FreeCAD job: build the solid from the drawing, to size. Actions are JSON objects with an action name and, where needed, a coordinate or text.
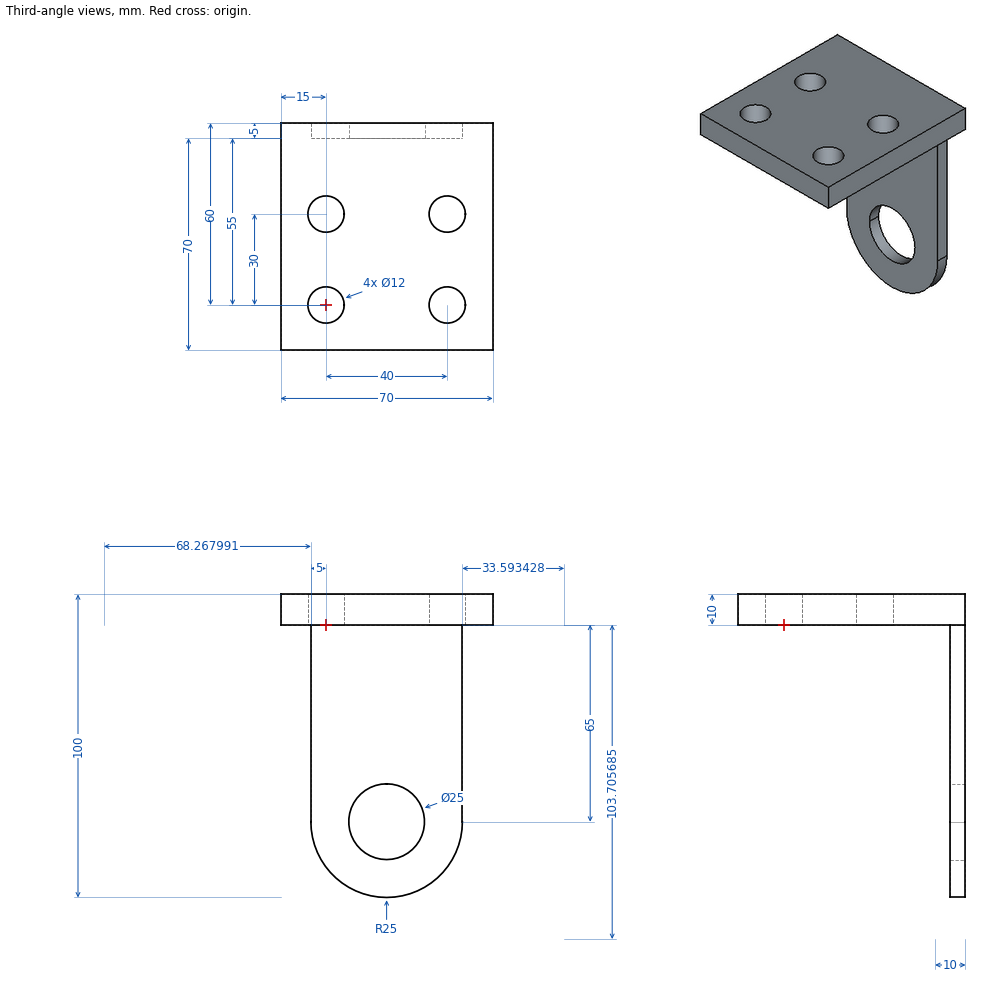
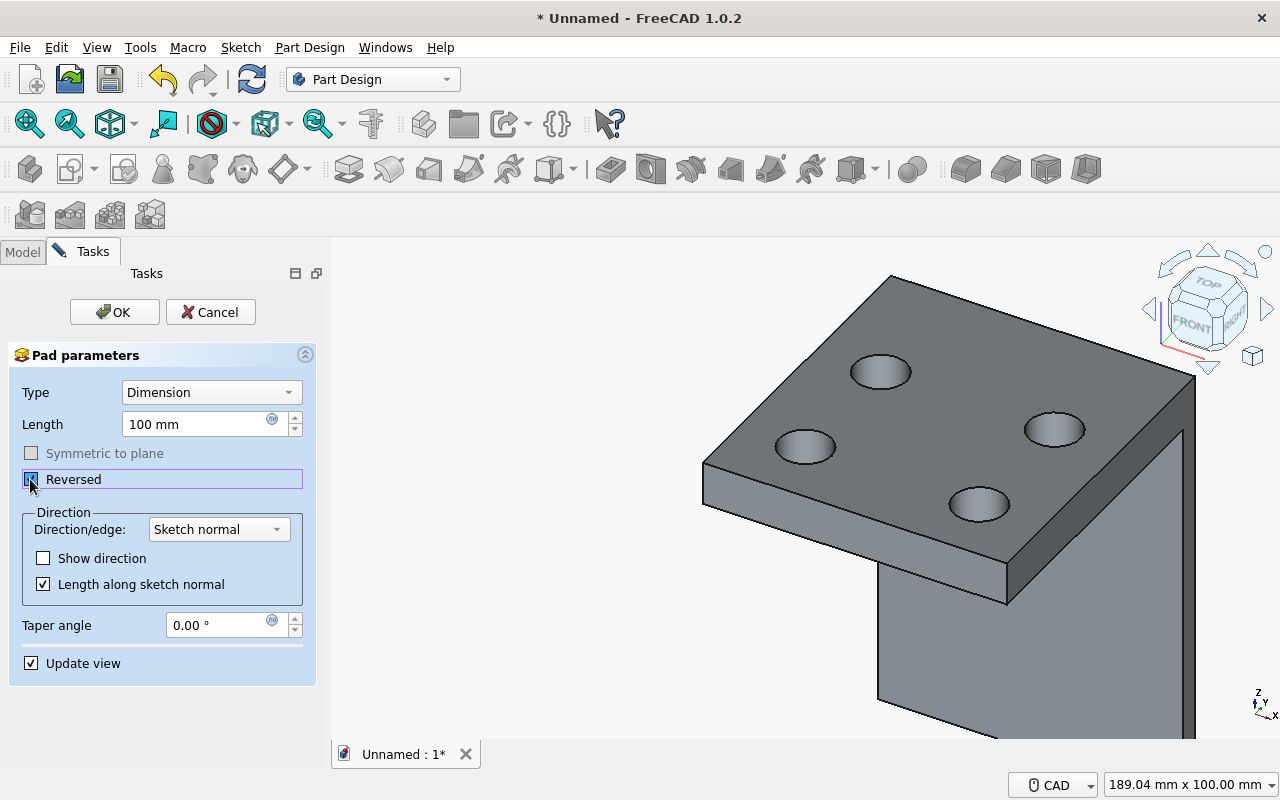
{"action": "left_click", "coordinate": [115, 312]}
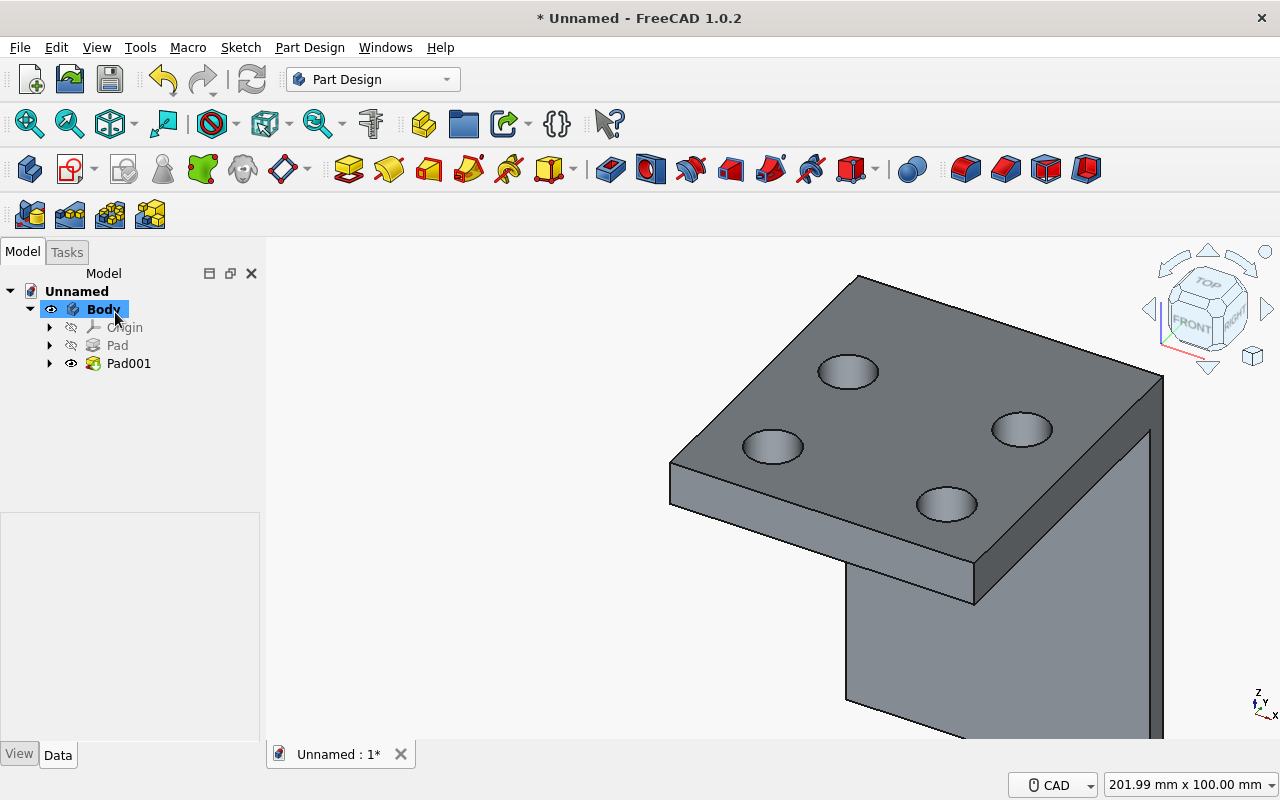
{"action": "left_click", "coordinate": [30, 124]}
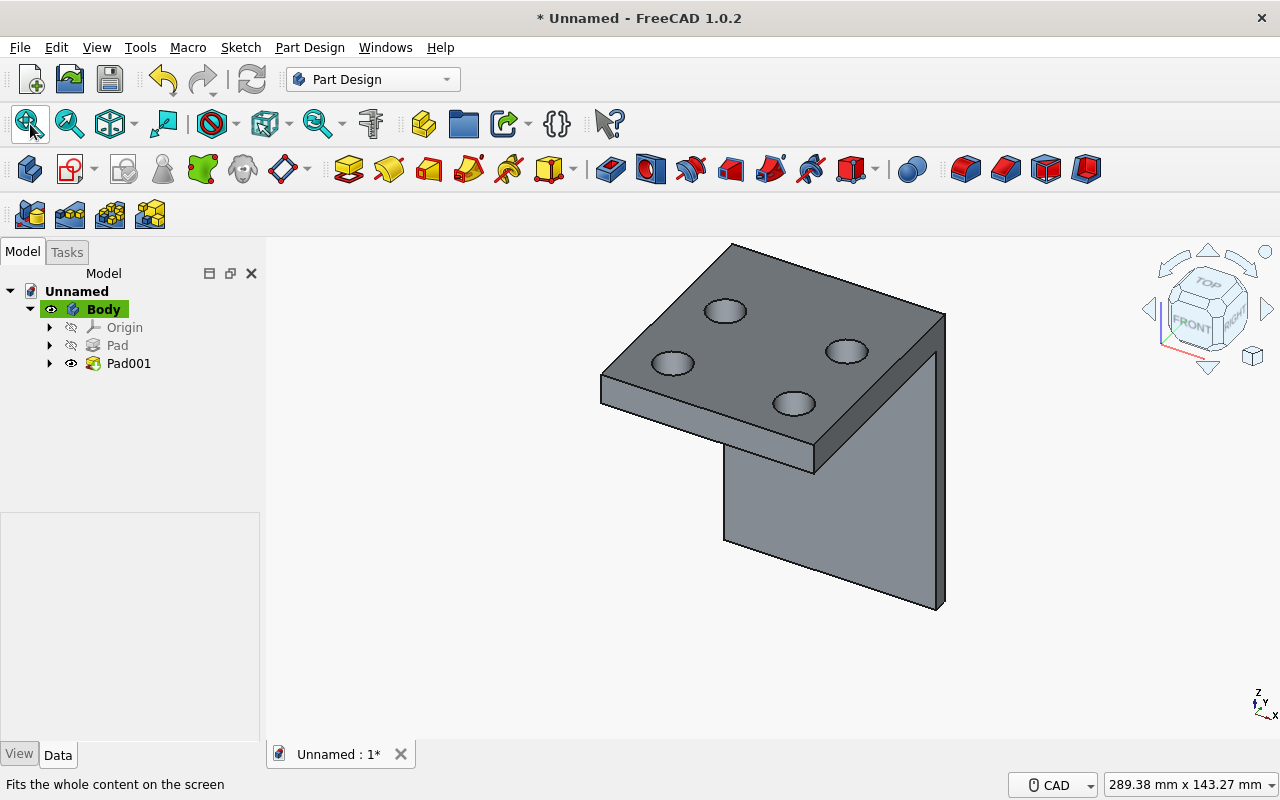
{"action": "key", "text": "4"}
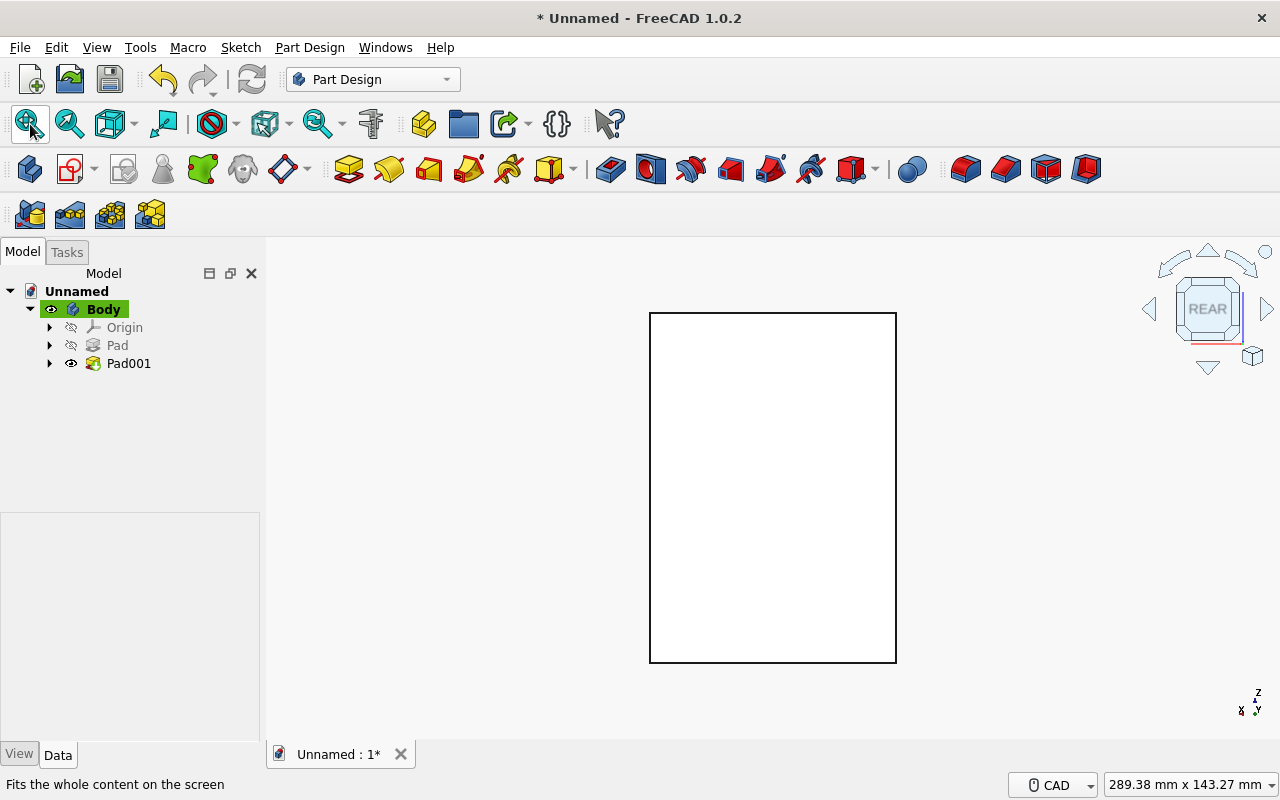
{"action": "left_click", "coordinate": [773, 437]}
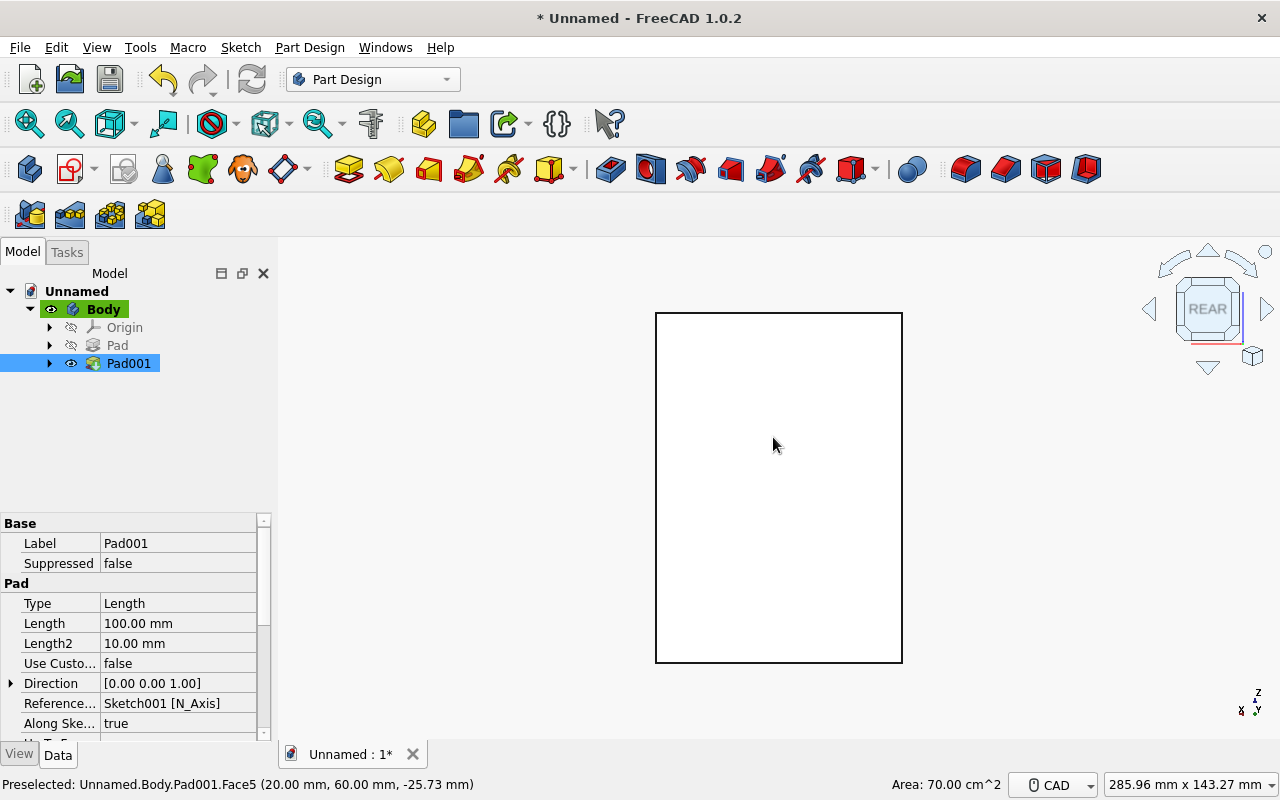
{"action": "left_click", "coordinate": [70, 170]}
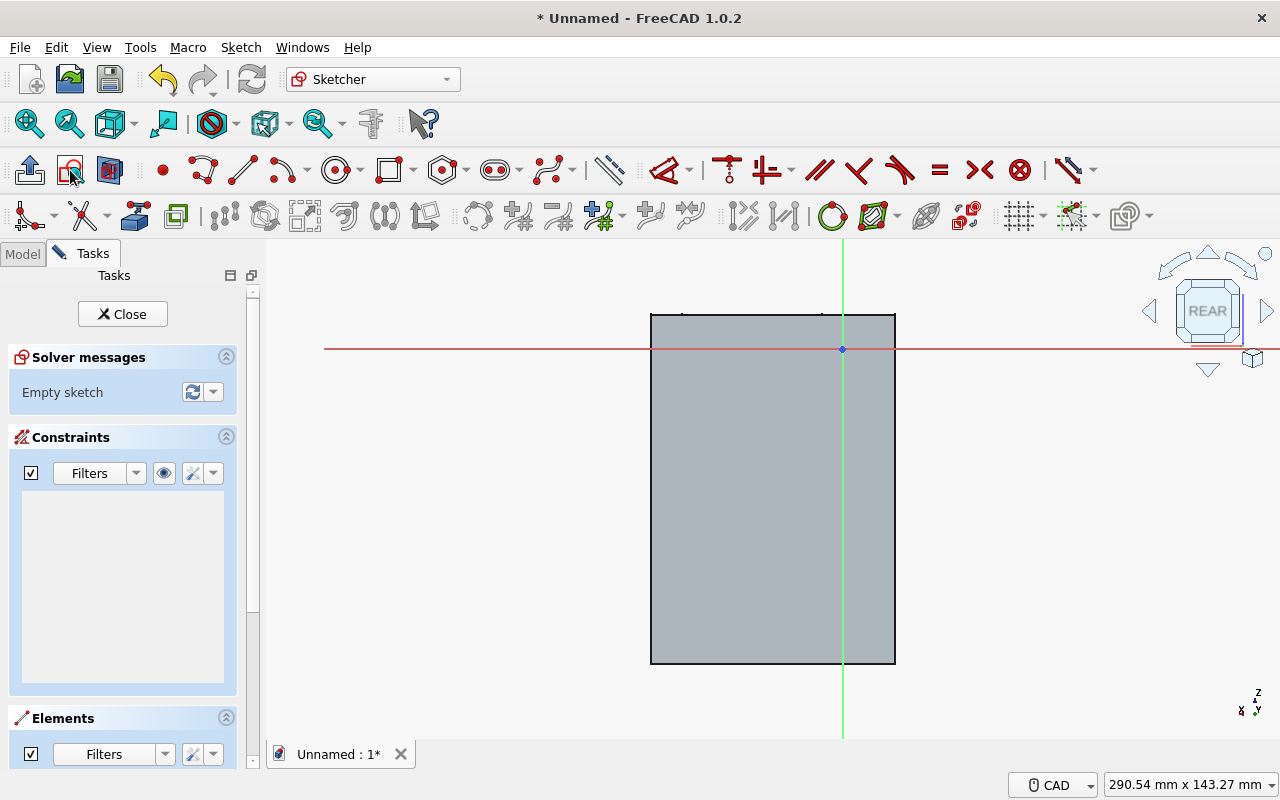
{"action": "scroll", "coordinate": [294, 302], "scroll_direction": "down", "scroll_amount": 1}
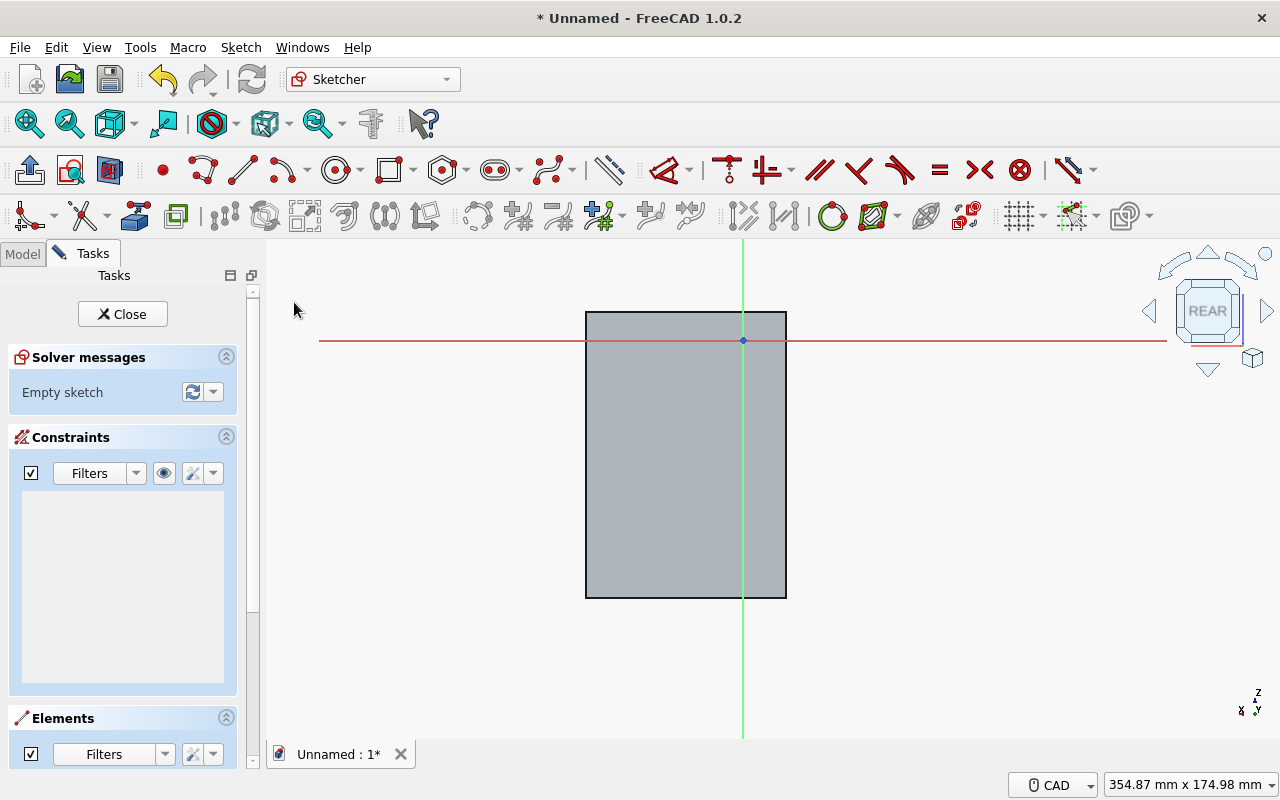
{"action": "left_click", "coordinate": [204, 170]}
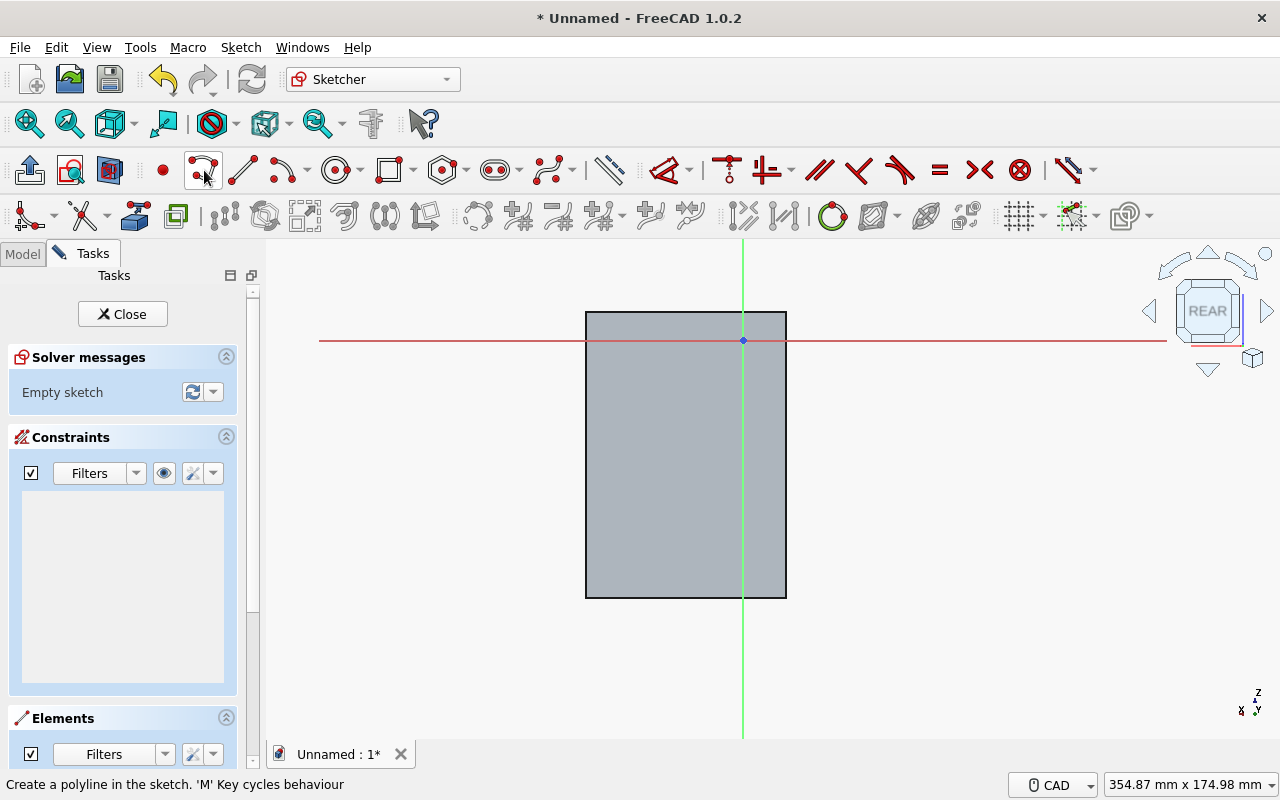
{"action": "left_click", "coordinate": [615, 527]}
{"action": "left_click", "coordinate": [615, 341]}
{"action": "left_click", "coordinate": [519, 350]}
{"action": "left_click", "coordinate": [519, 637]}
{"action": "left_click", "coordinate": [953, 637]}
{"action": "left_click", "coordinate": [953, 341]}
{"action": "left_click", "coordinate": [758, 350]}
{"action": "left_click", "coordinate": [758, 527]}
{"action": "right_click", "coordinate": [758, 527]}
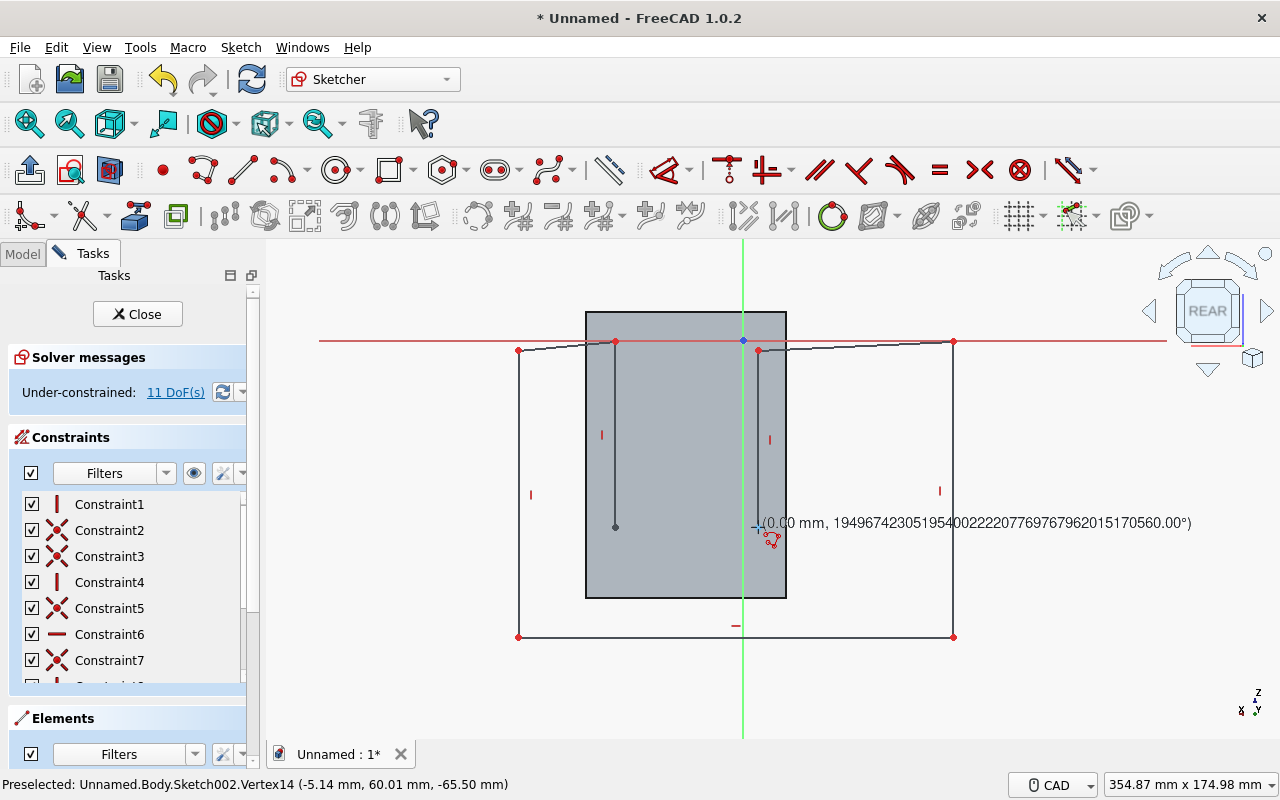
{"action": "key", "text": "g 3 a"}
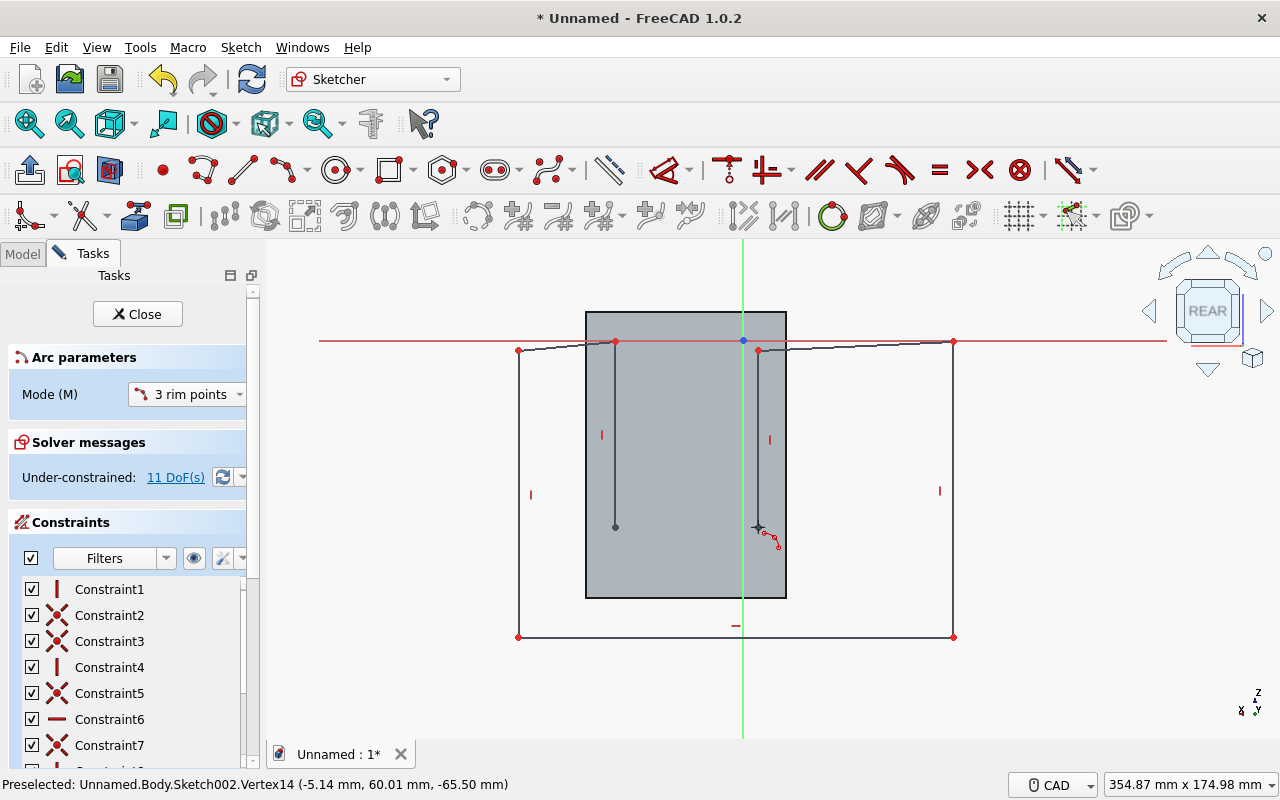
{"action": "left_click", "coordinate": [758, 528]}
{"action": "left_click", "coordinate": [615, 528]}
{"action": "left_click", "coordinate": [686, 598]}